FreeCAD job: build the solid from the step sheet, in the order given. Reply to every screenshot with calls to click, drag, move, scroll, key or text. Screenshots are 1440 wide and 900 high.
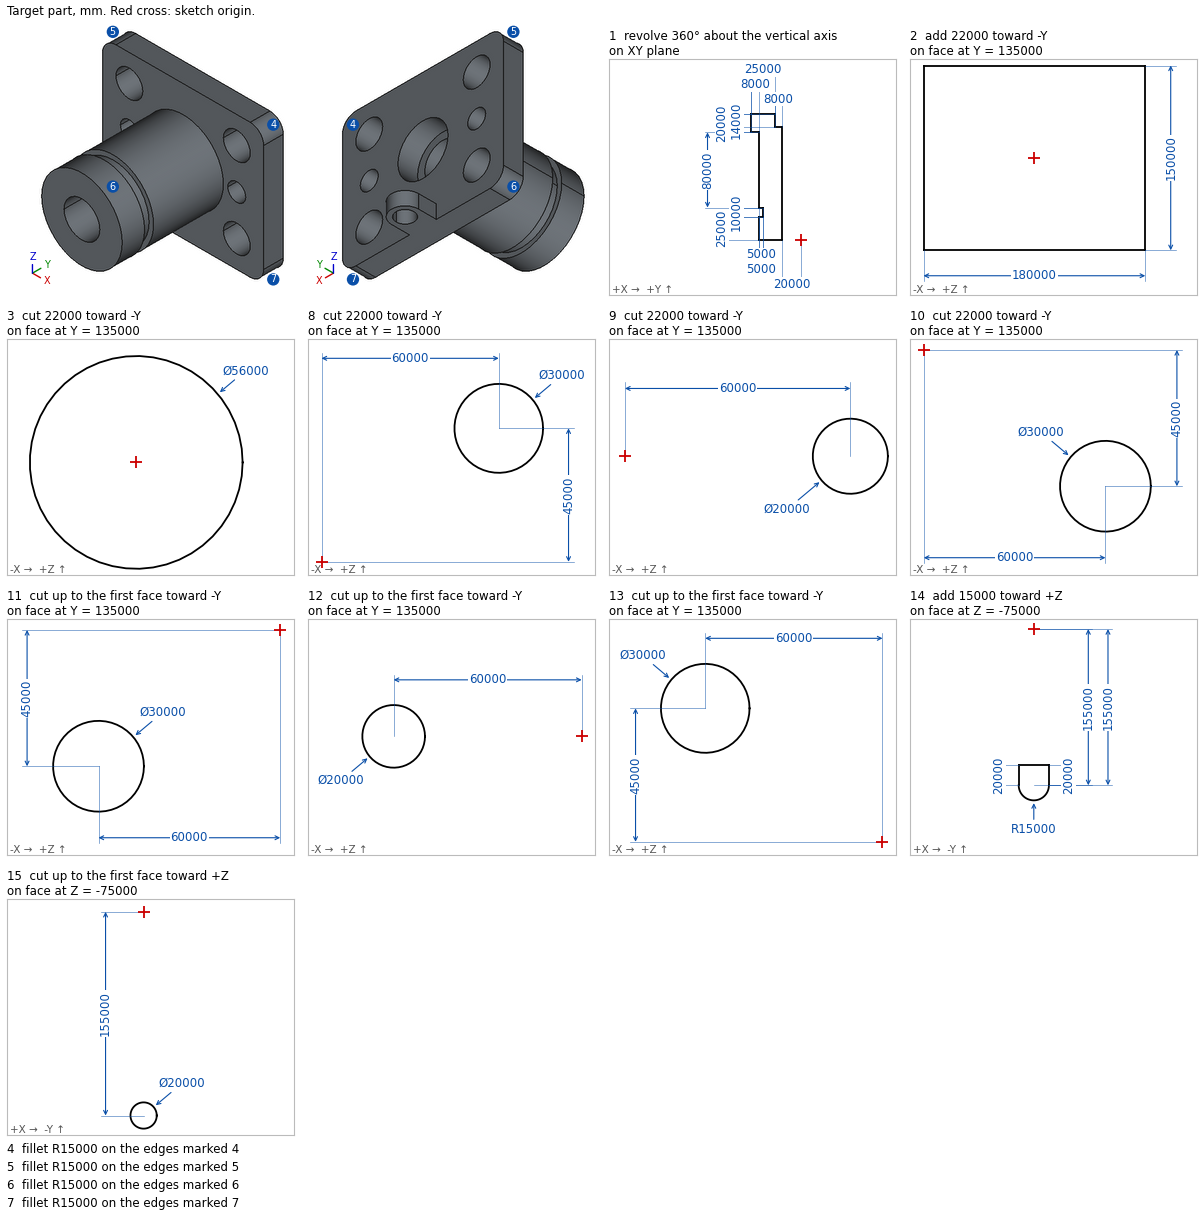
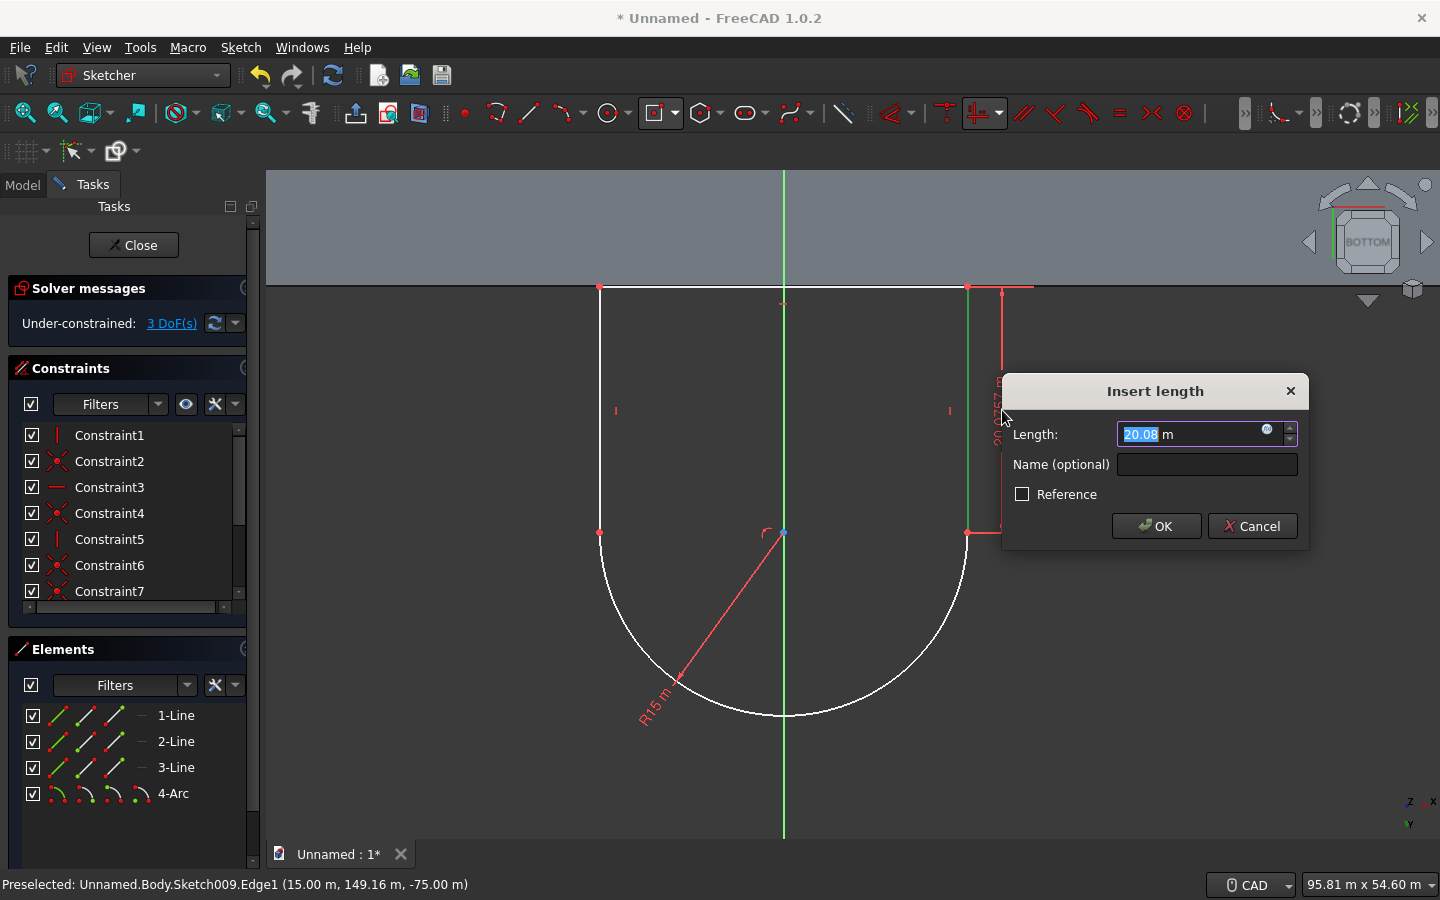
key(ctrl+a)
text(20000 mm)
key(Return)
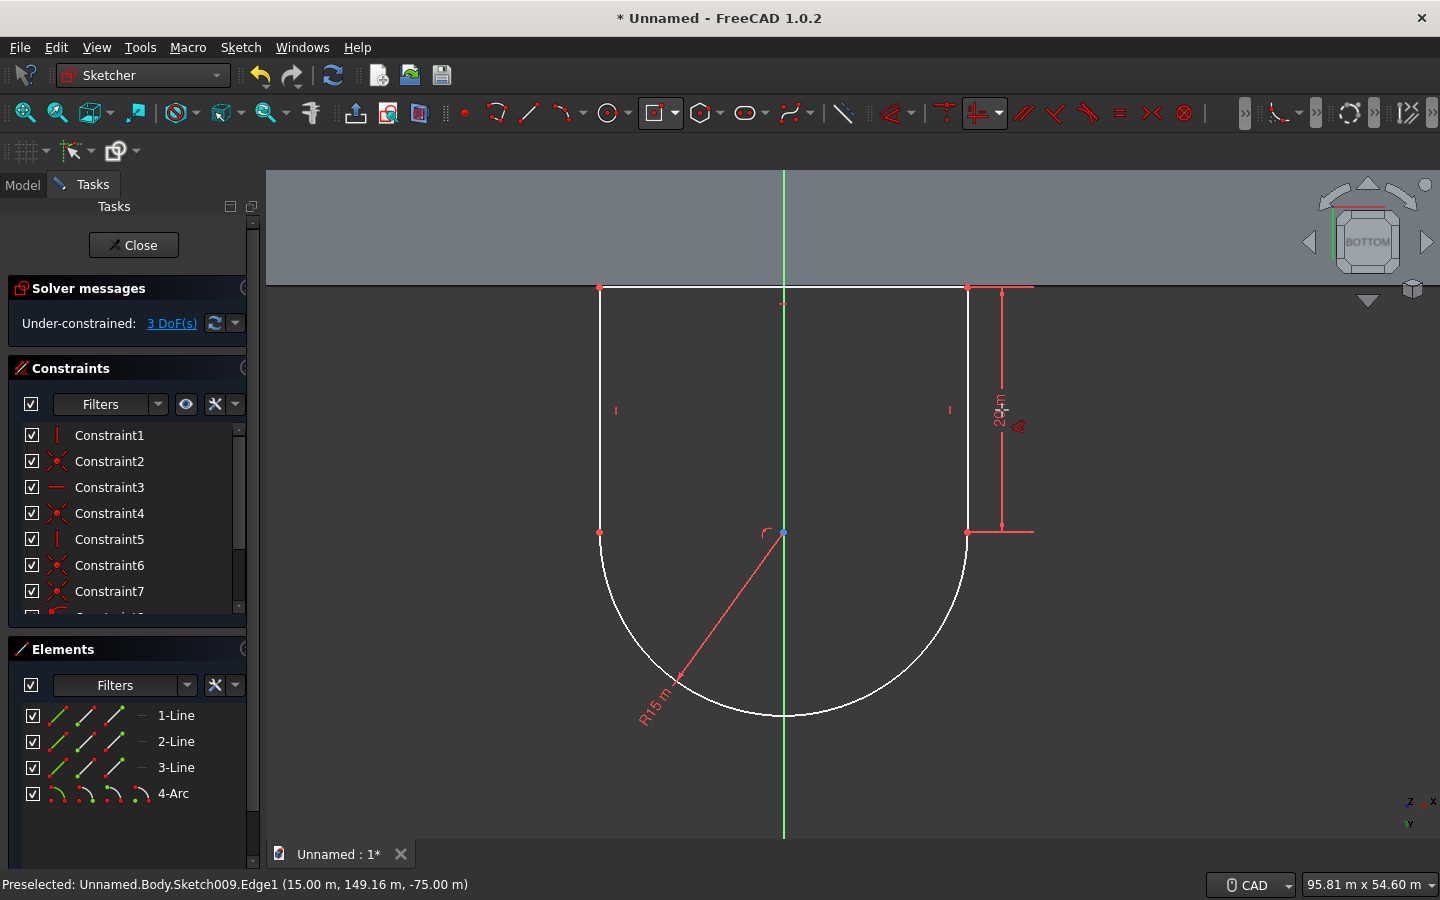
click(600, 361)
click(566, 410)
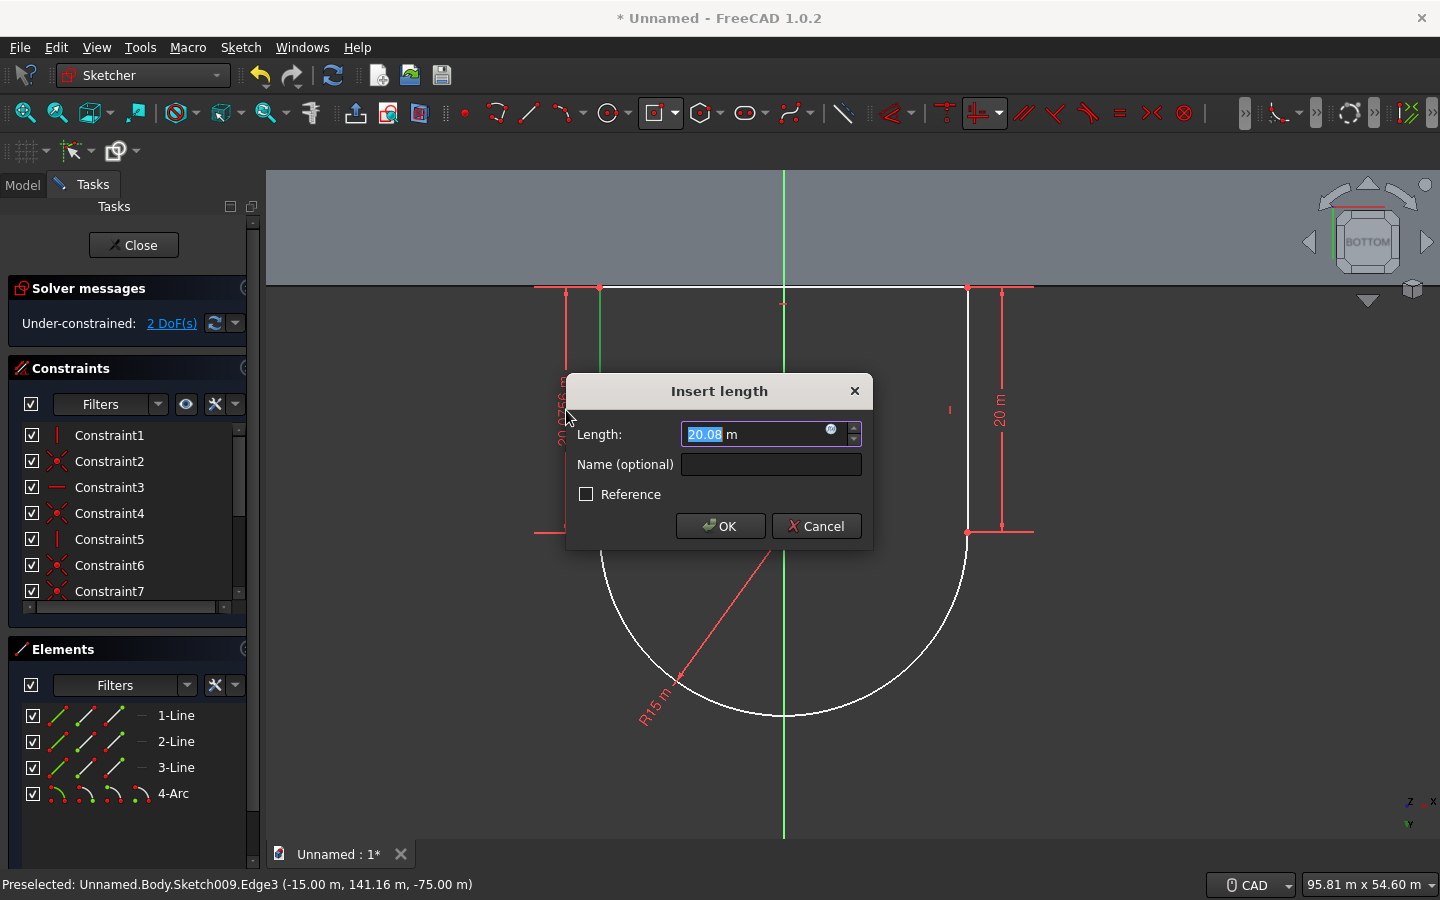
key(ctrl+a)
text(20000 mm)
key(Return)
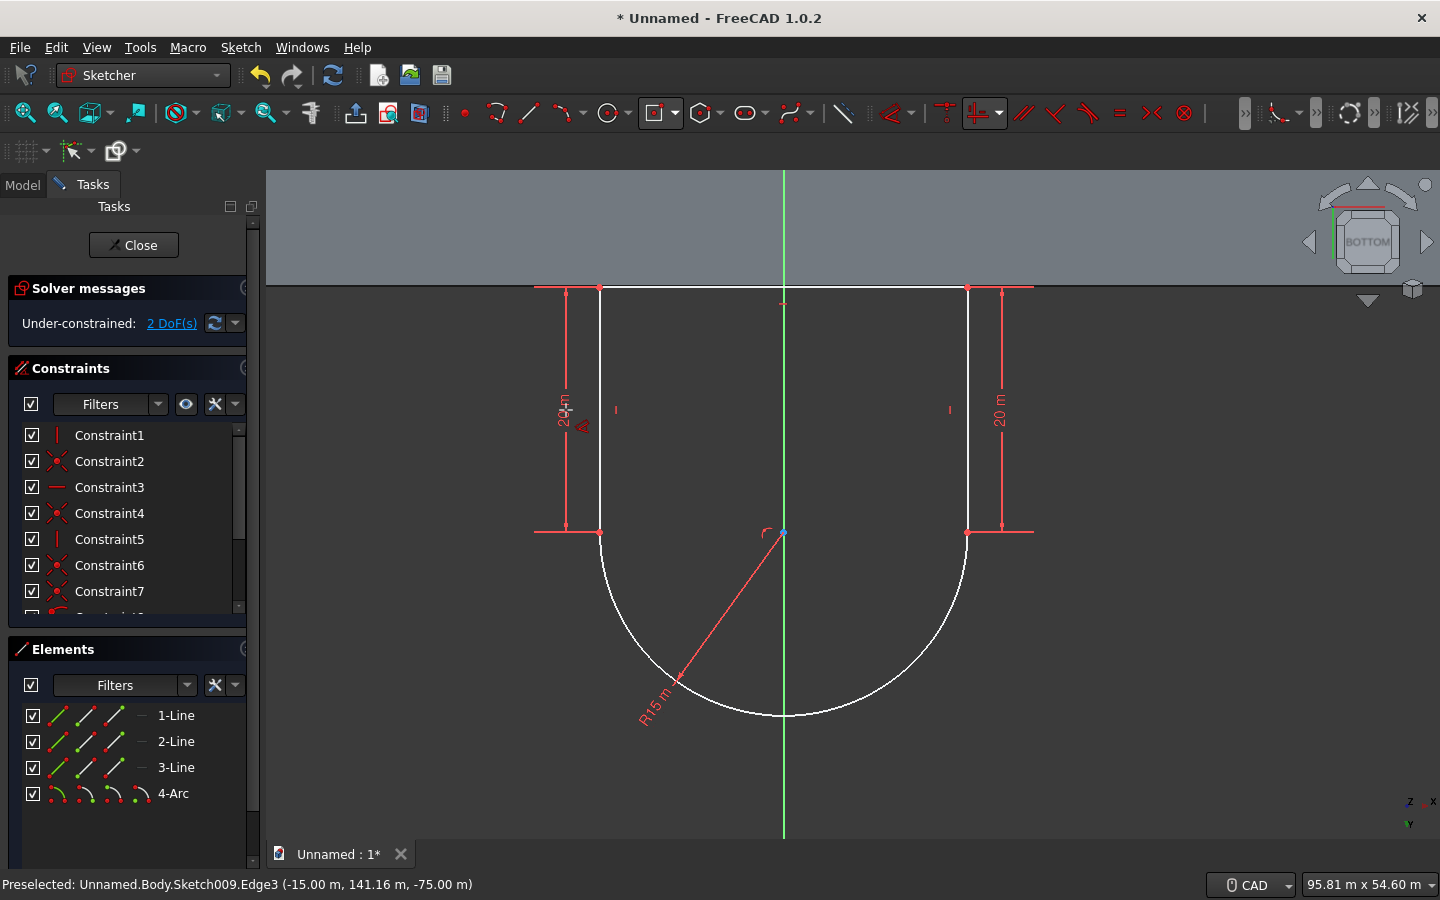
click(968, 532)
click(1002, 365)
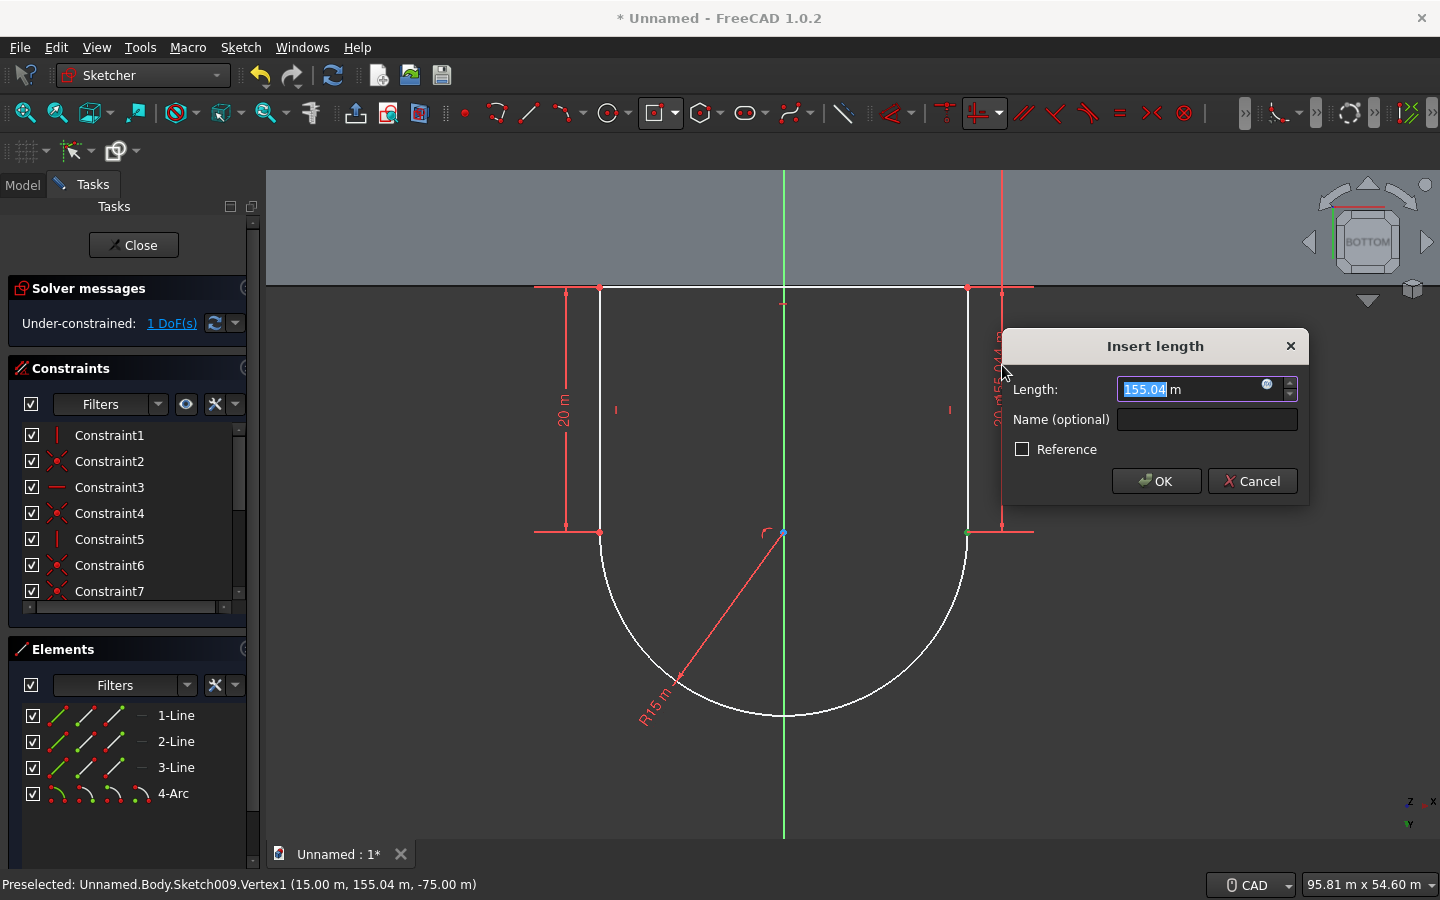
key(ctrl+a)
text(155000 mm)
key(Return)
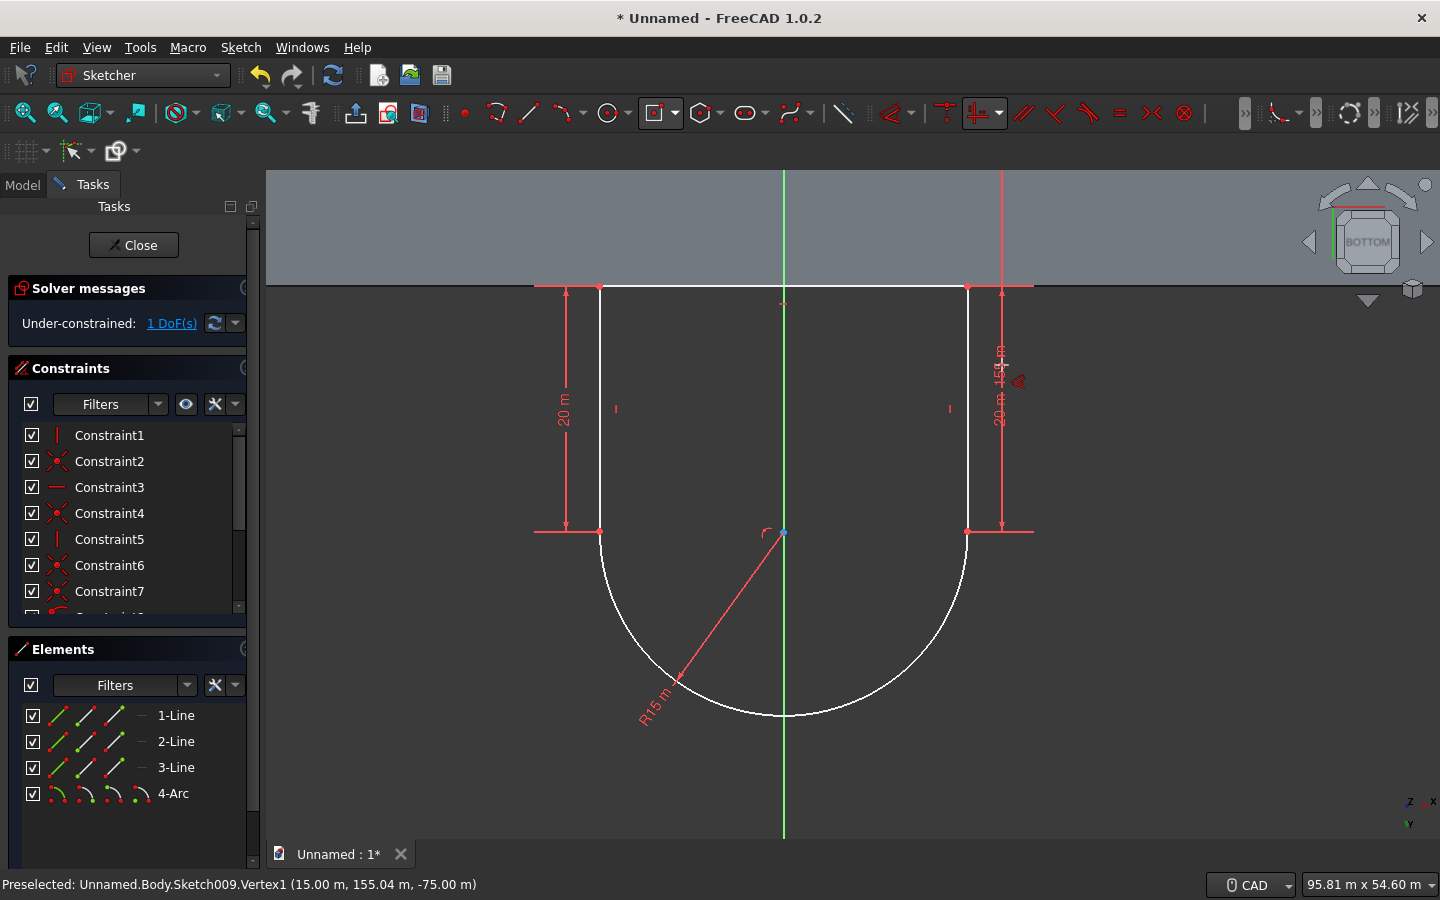
click(784, 532)
click(818, 365)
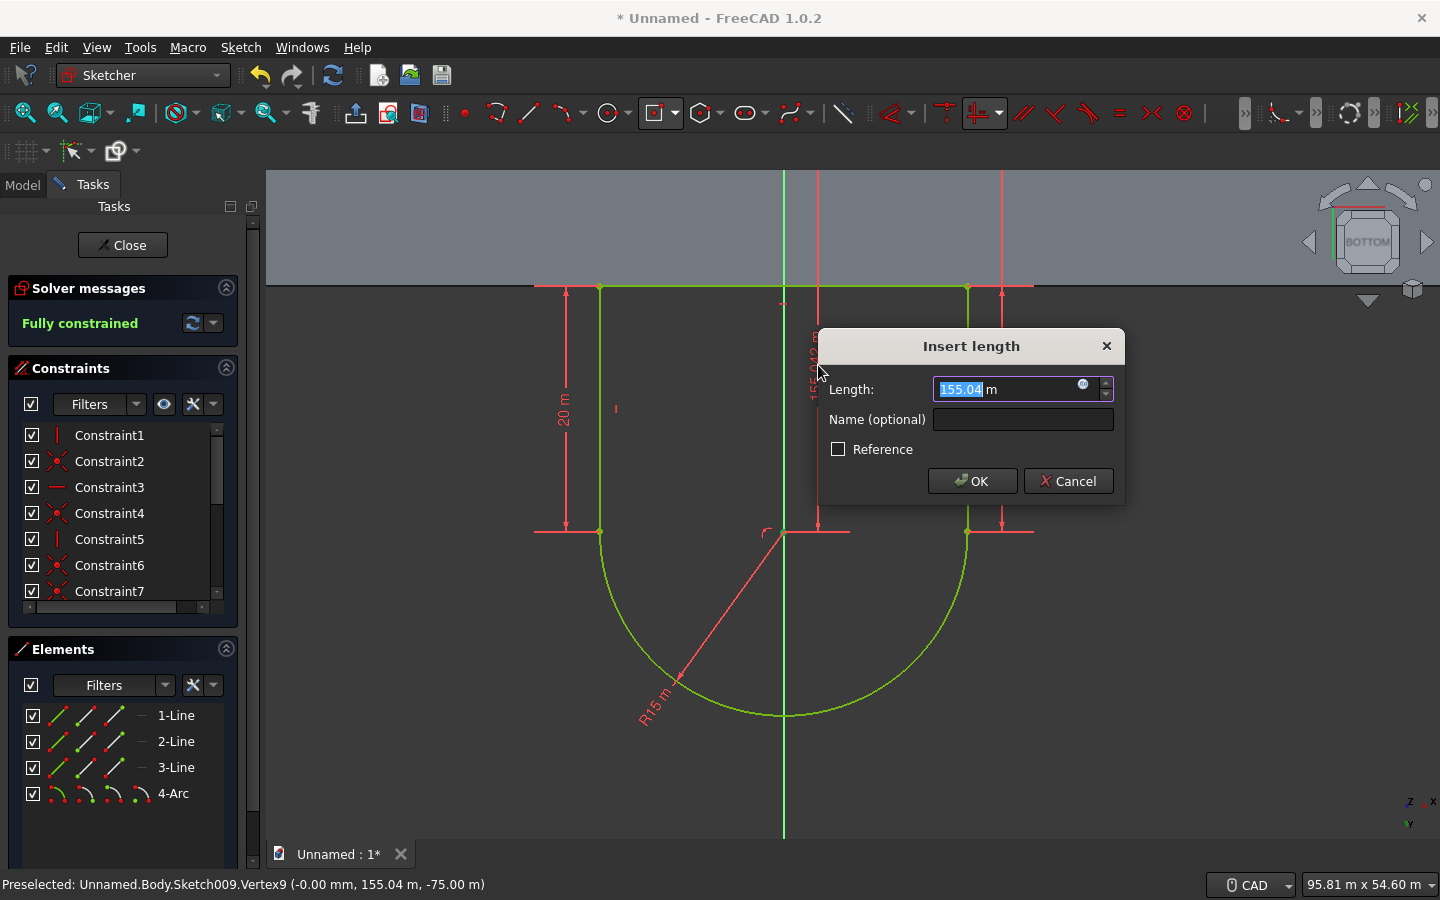
key(ctrl+a)
text(155000 mm)
key(Return)
key(Escape)